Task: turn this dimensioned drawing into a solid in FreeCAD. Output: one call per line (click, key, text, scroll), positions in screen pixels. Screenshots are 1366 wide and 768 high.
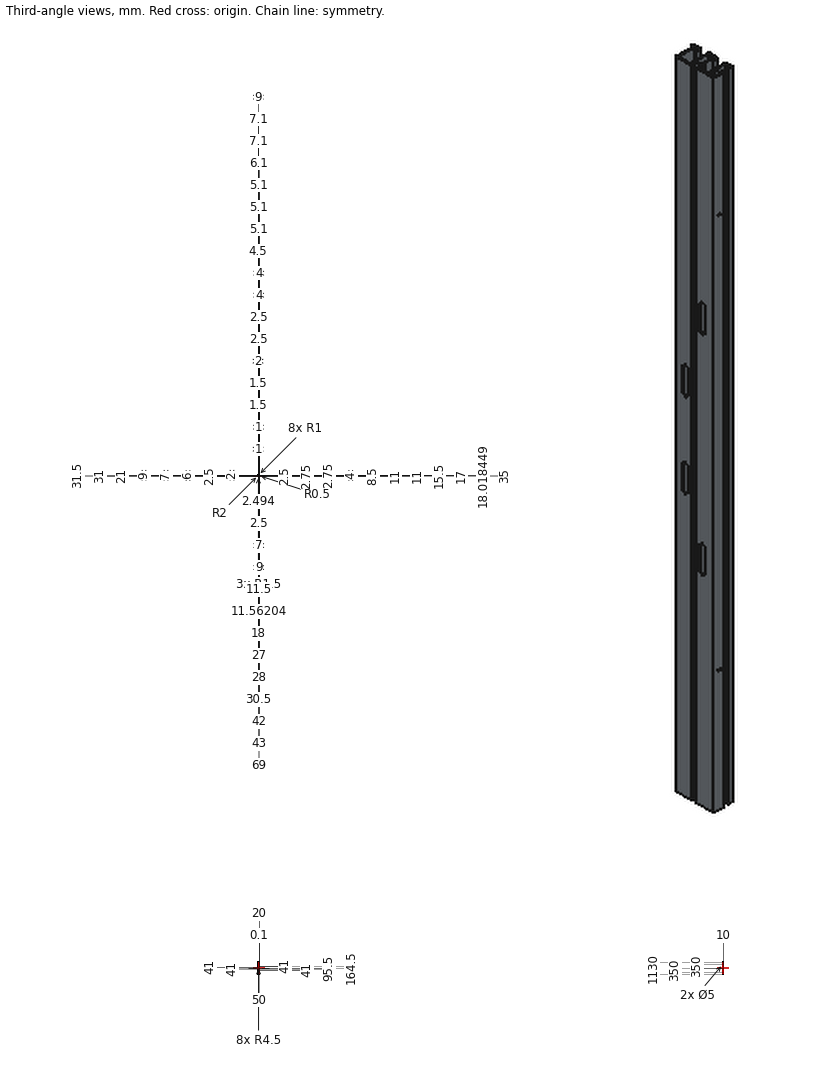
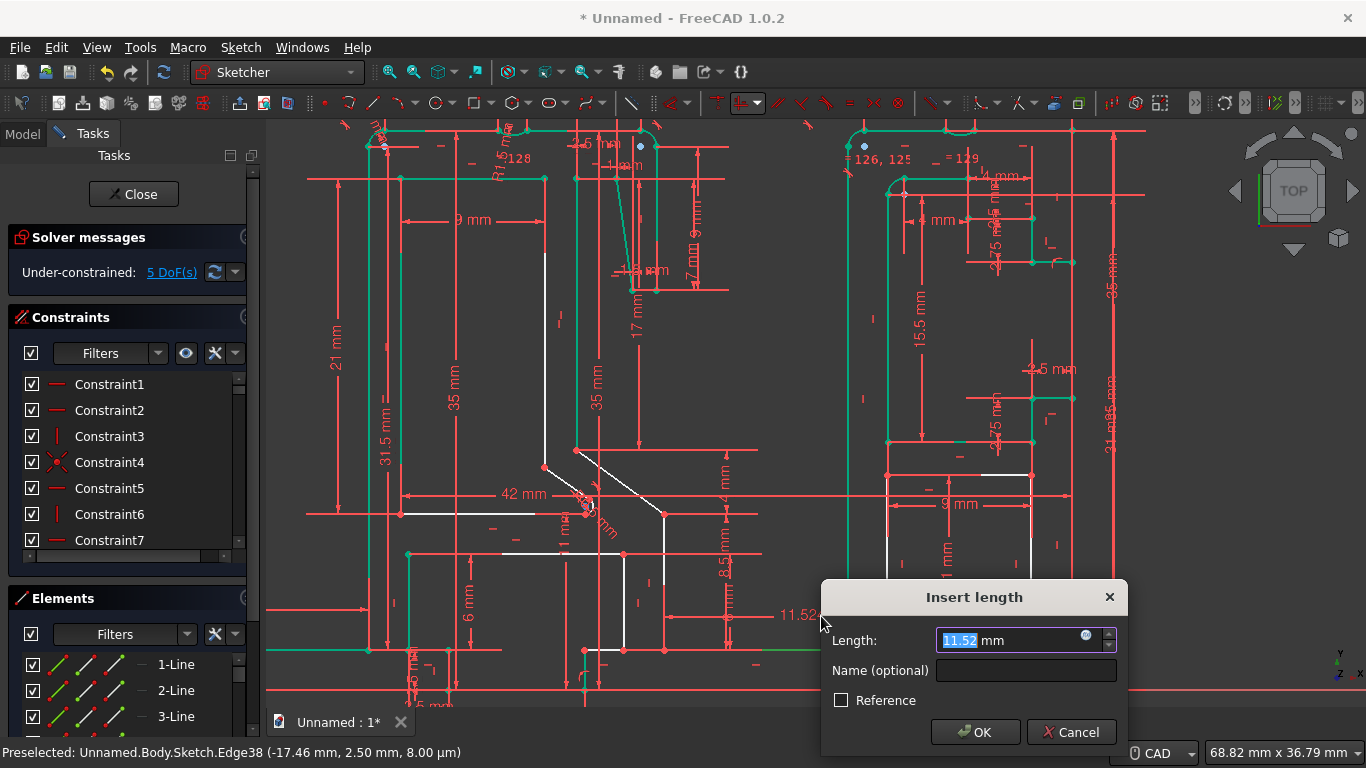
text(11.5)
key(Return)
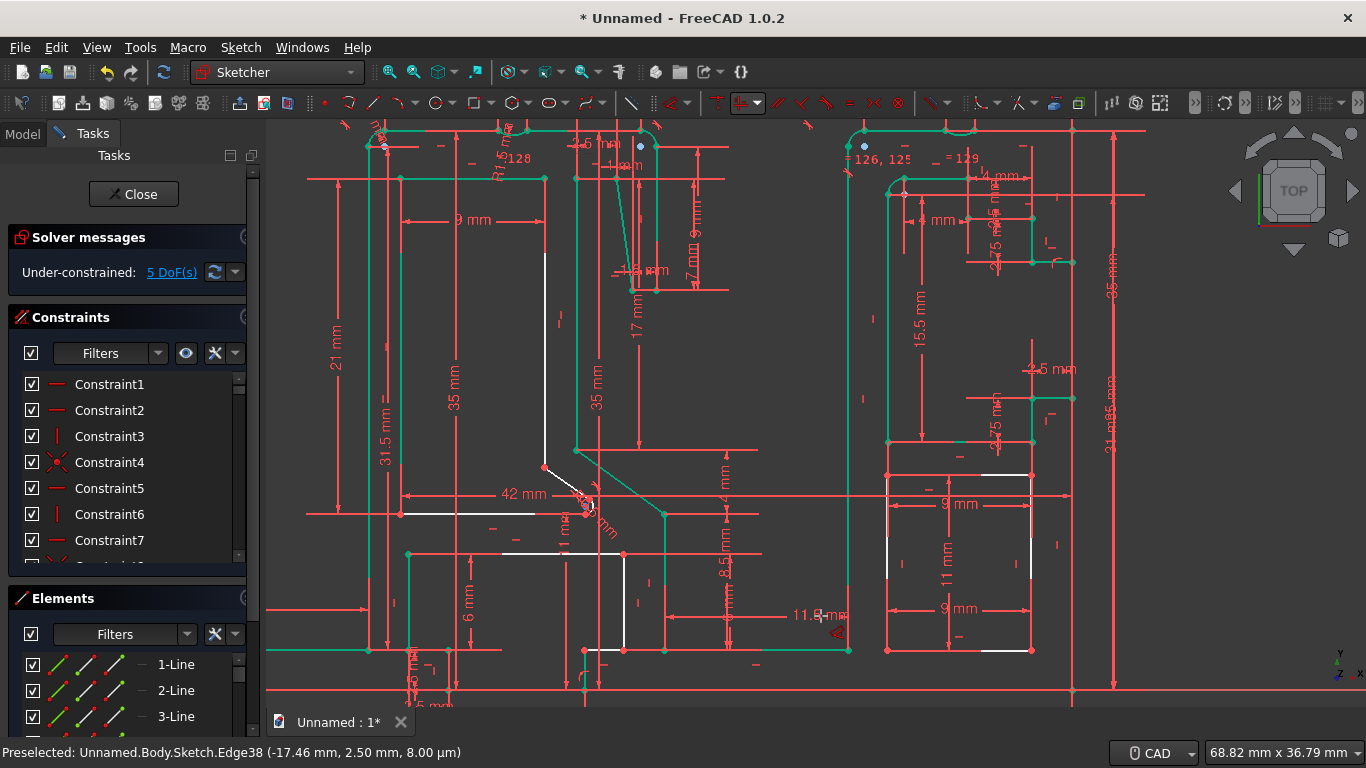
click(887, 651)
click(1106, 665)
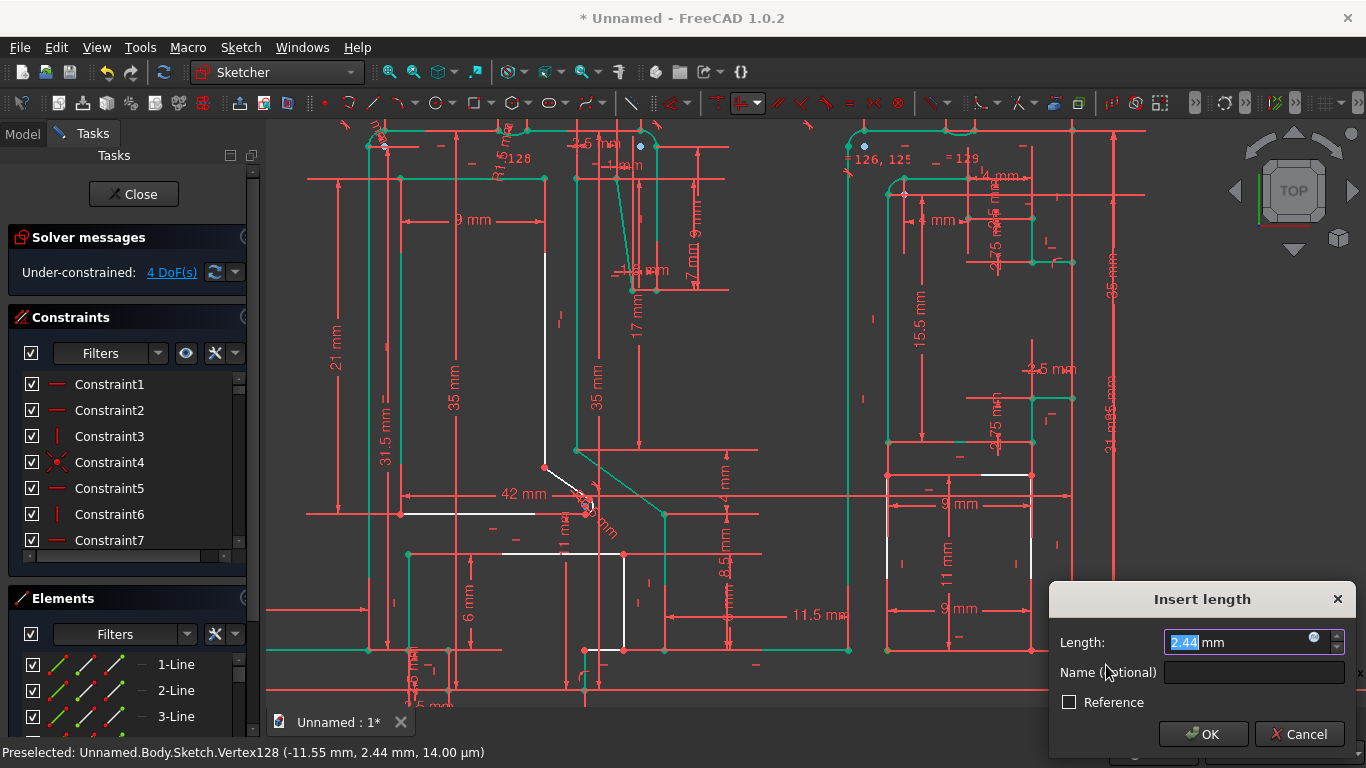
text(2.5)
key(Return)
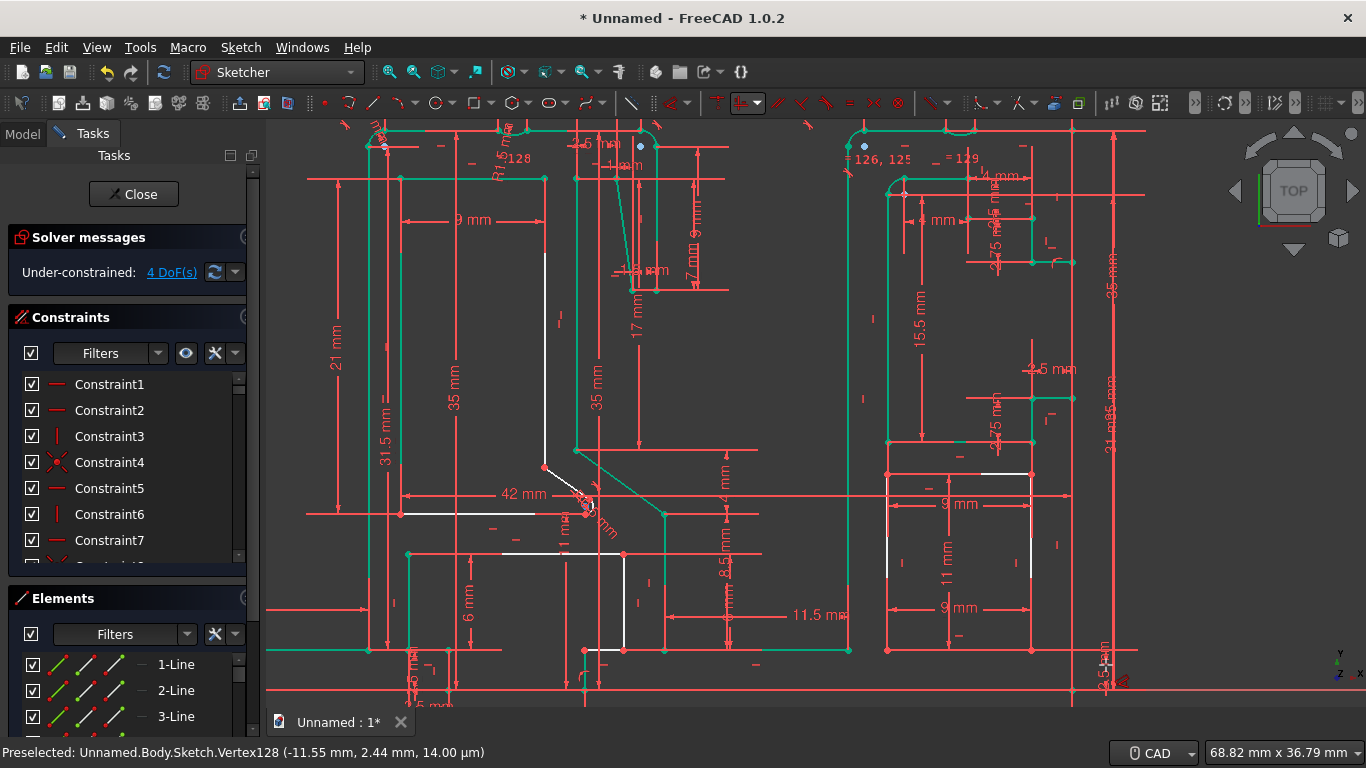
click(1031, 650)
click(1052, 616)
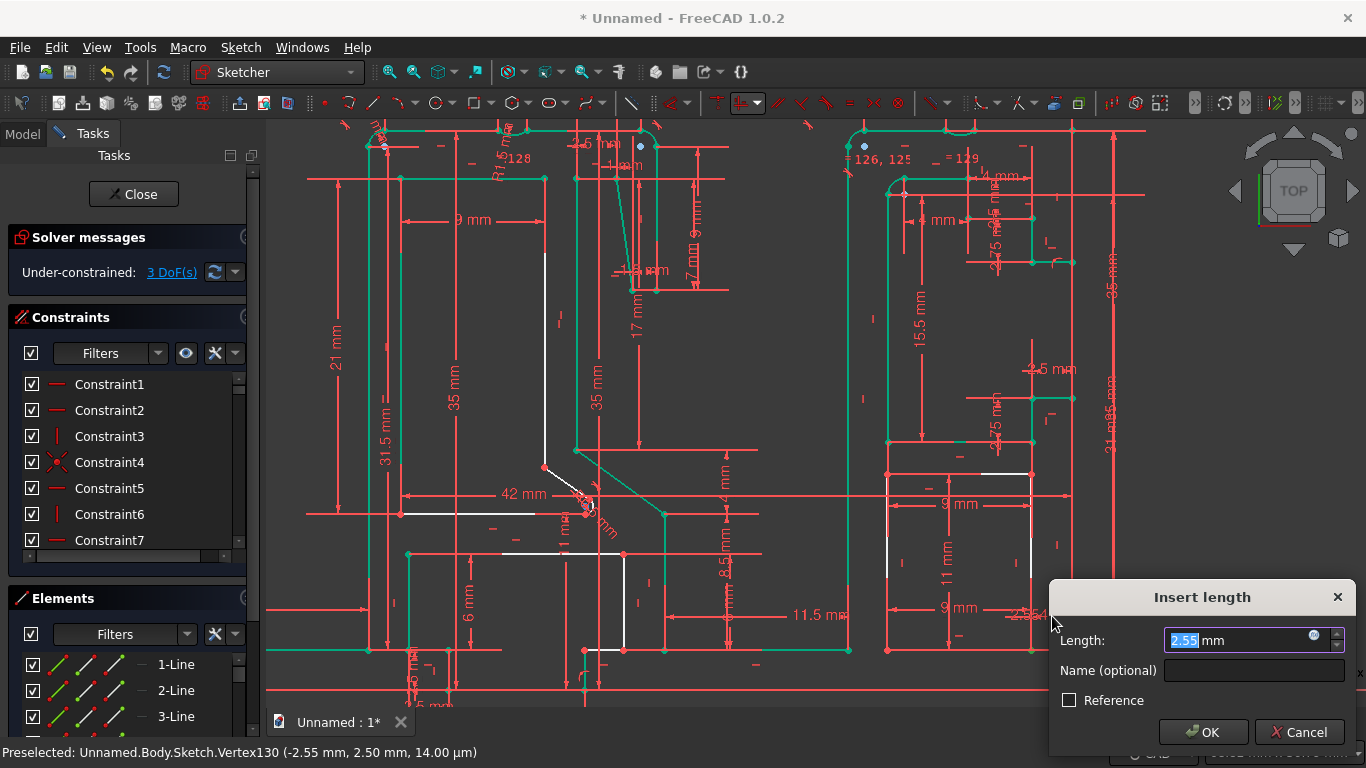
text(2.5)
key(Return)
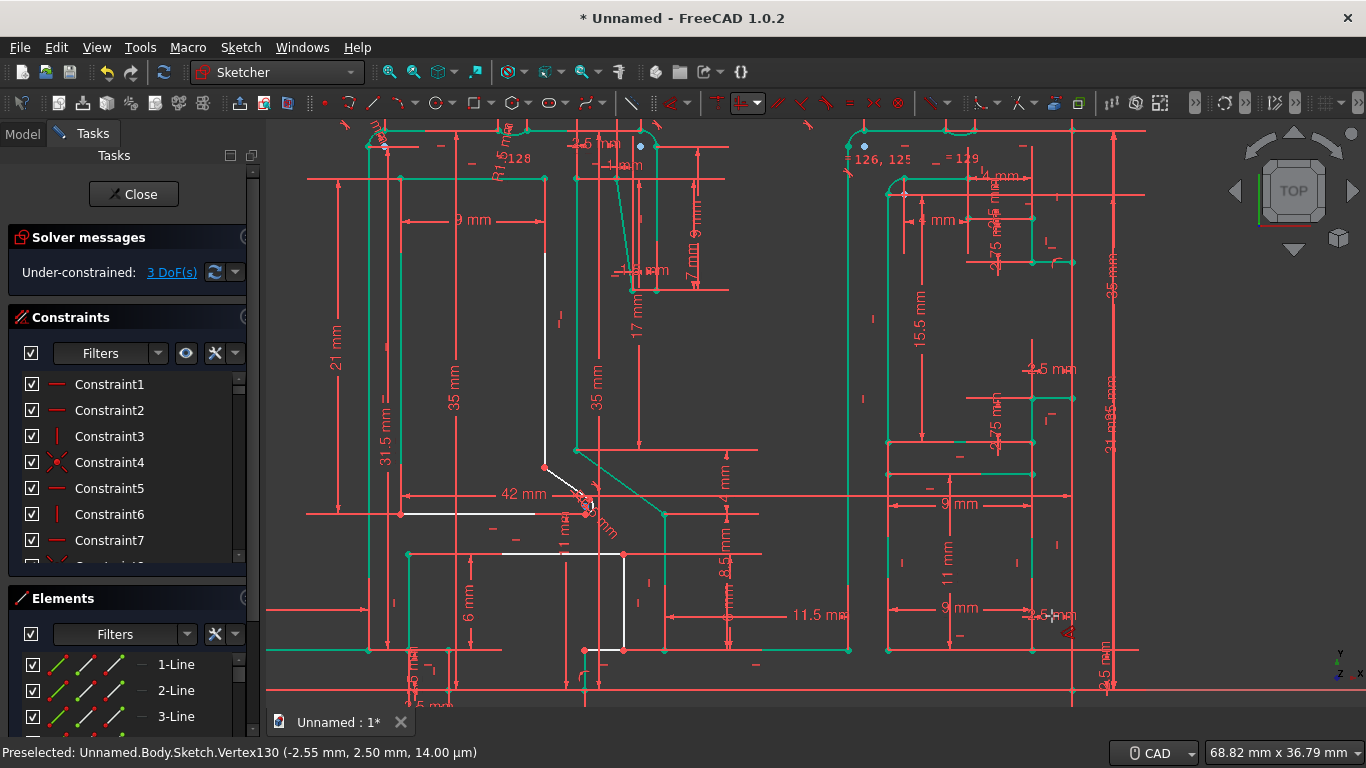
click(612, 650)
click(604, 616)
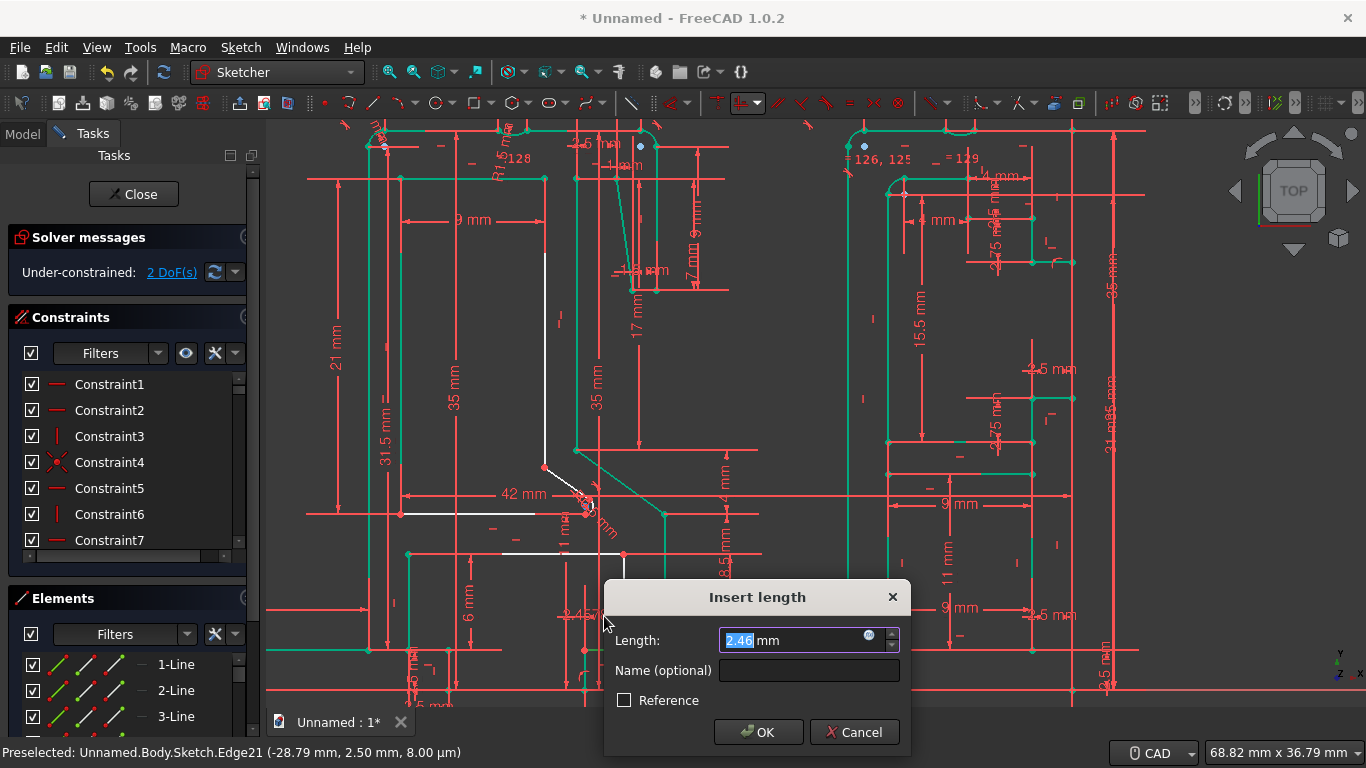
text(2.494)
key(Return)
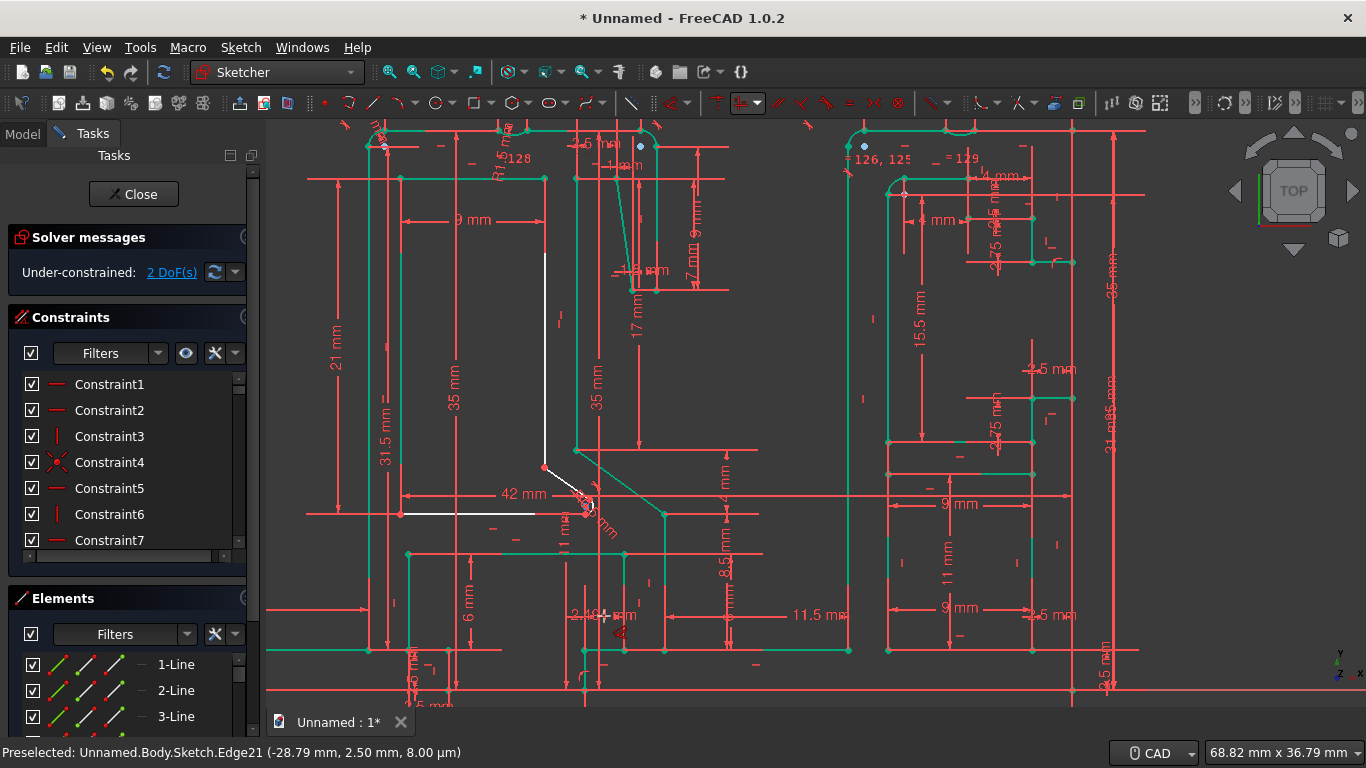
click(530, 514)
click(451, 480)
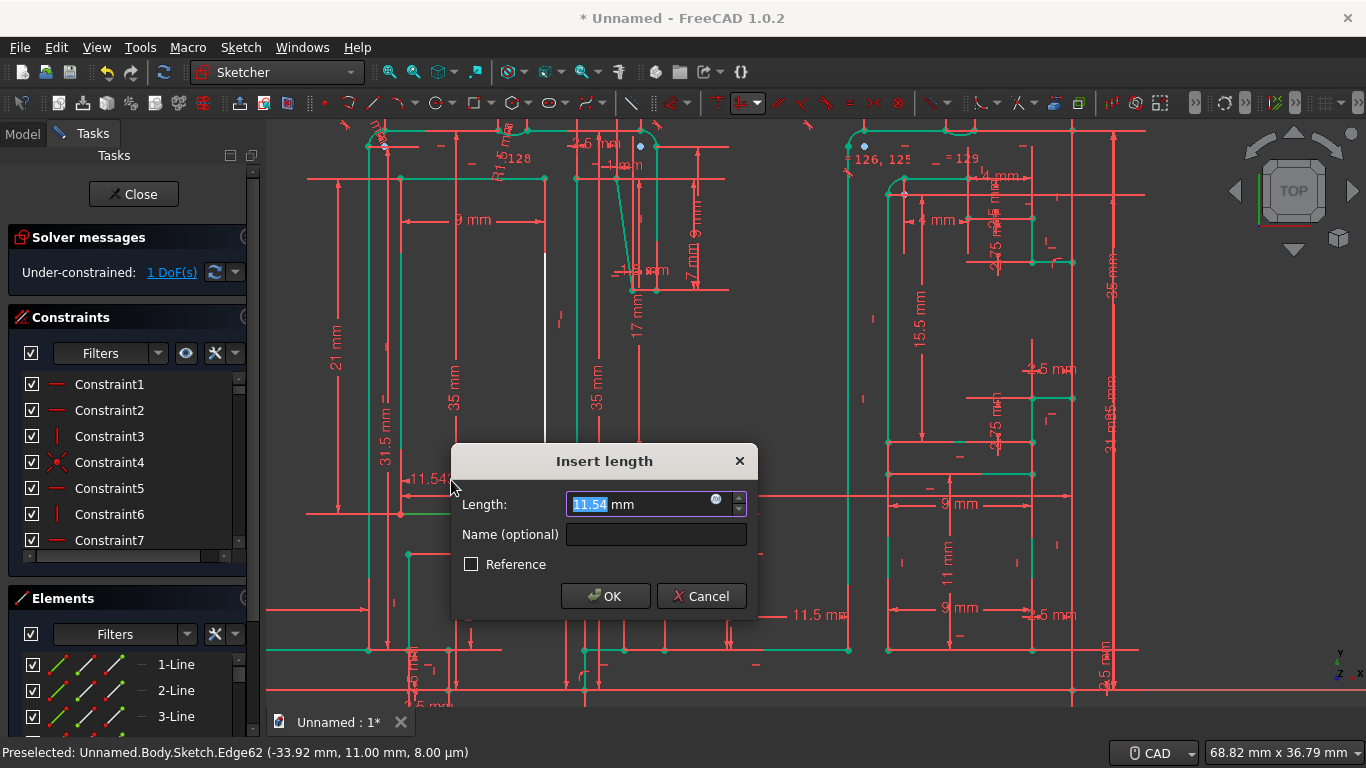
text(11.56204)
key(Return)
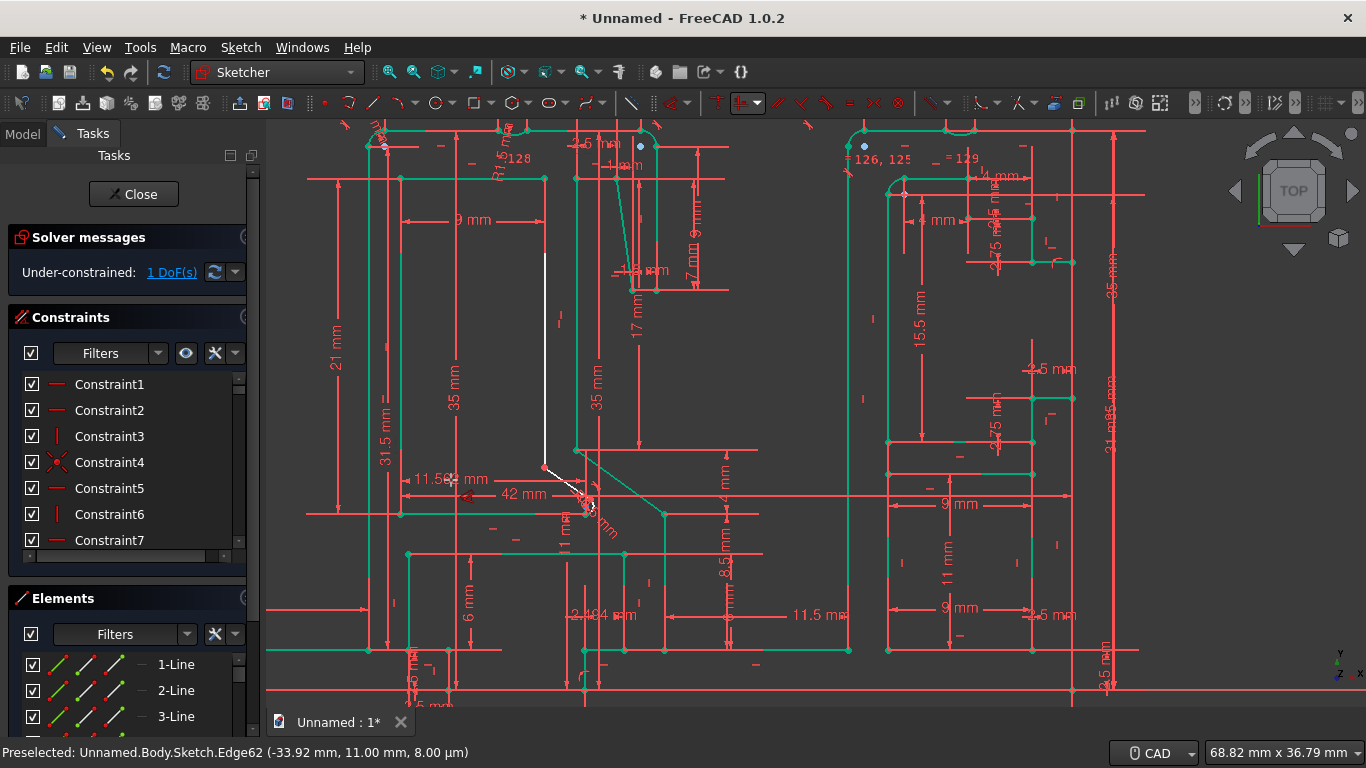
click(545, 265)
click(511, 323)